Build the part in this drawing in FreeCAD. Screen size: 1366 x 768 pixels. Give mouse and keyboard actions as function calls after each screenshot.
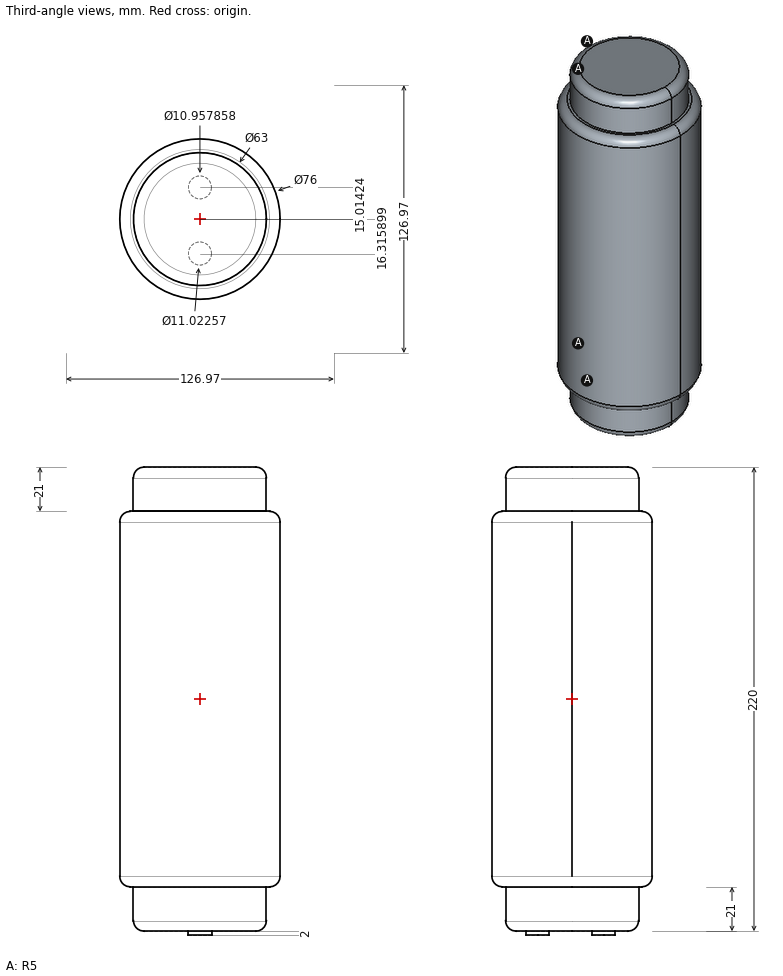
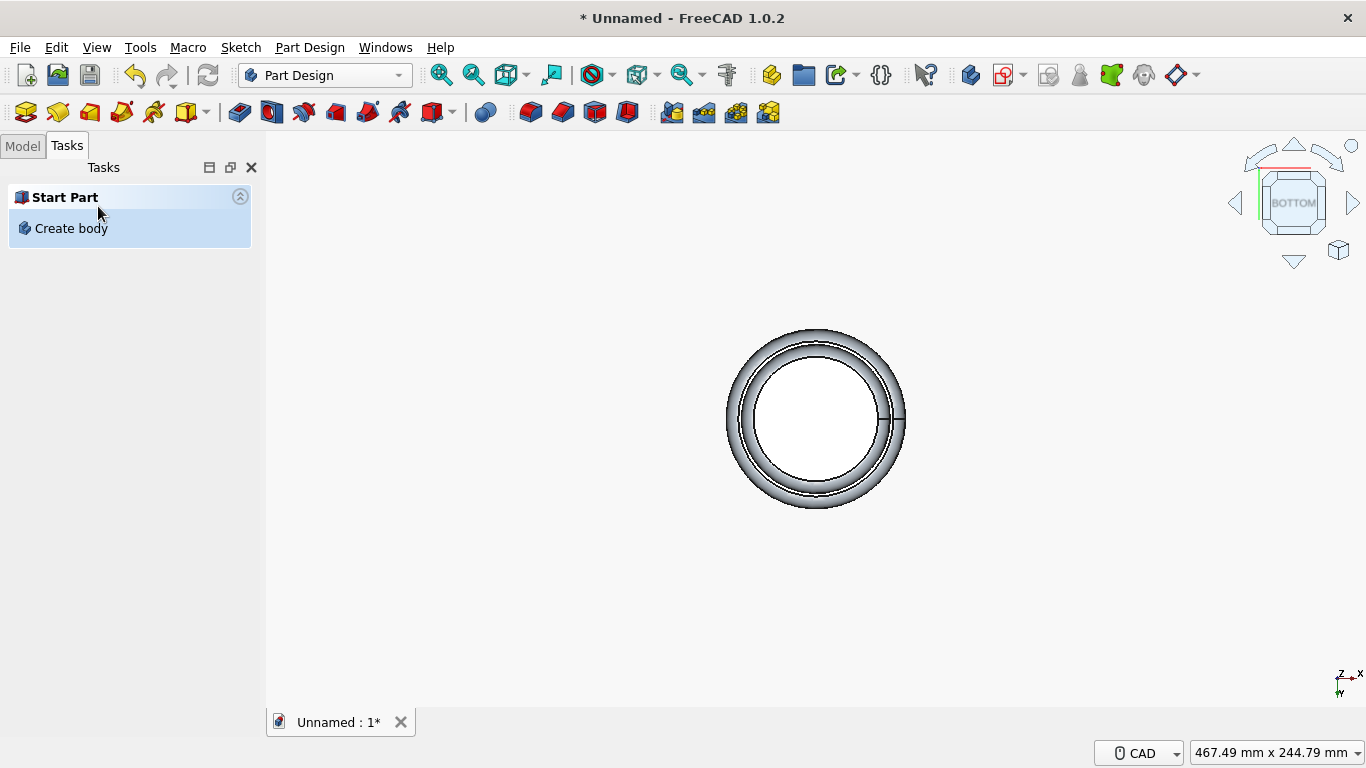
key(v)
key(f)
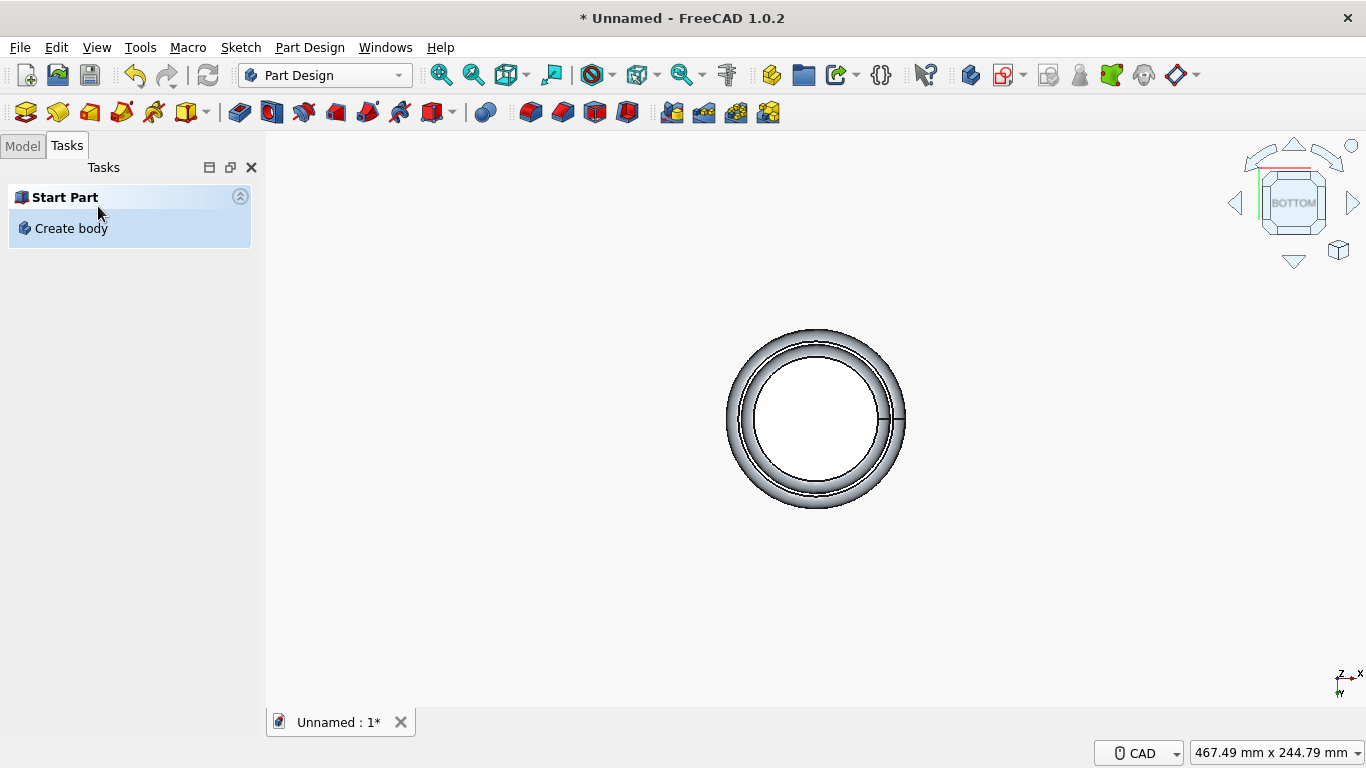
click(816, 418)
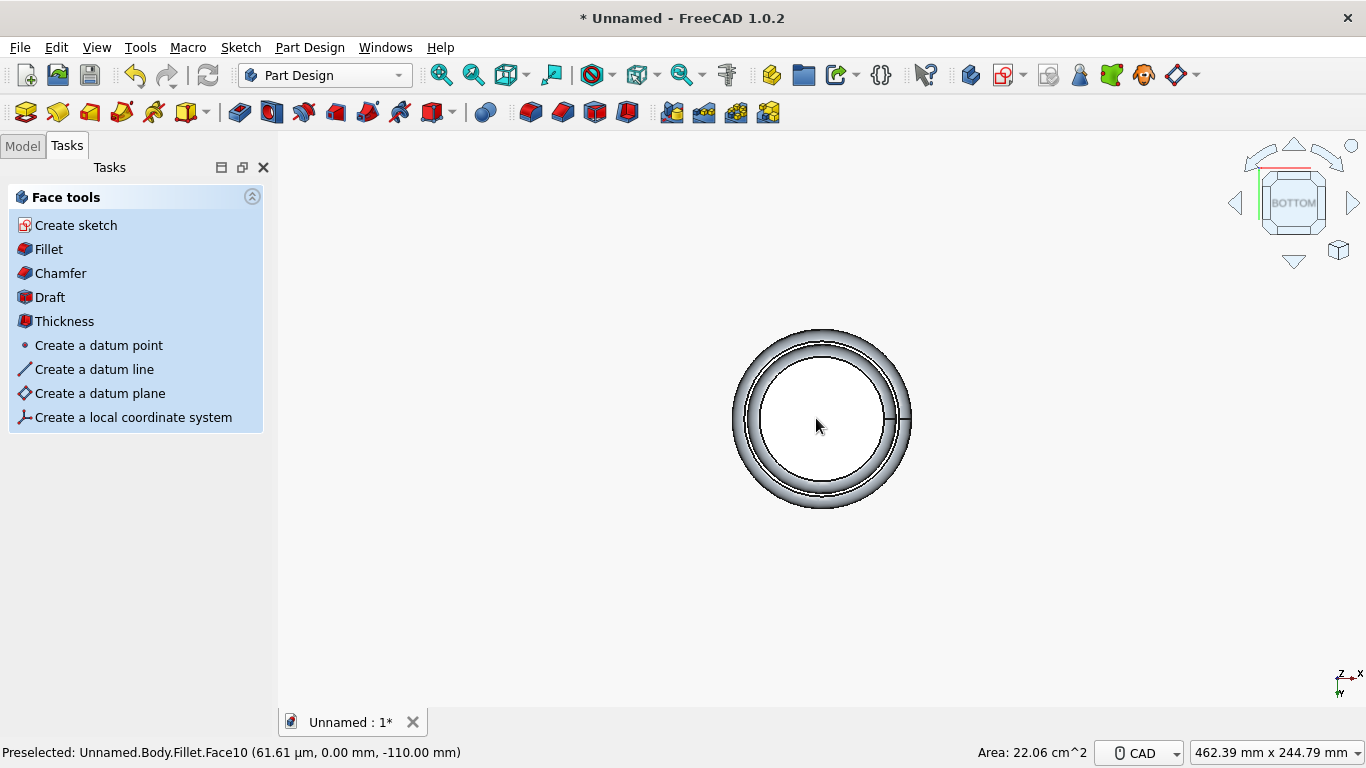
click(1004, 76)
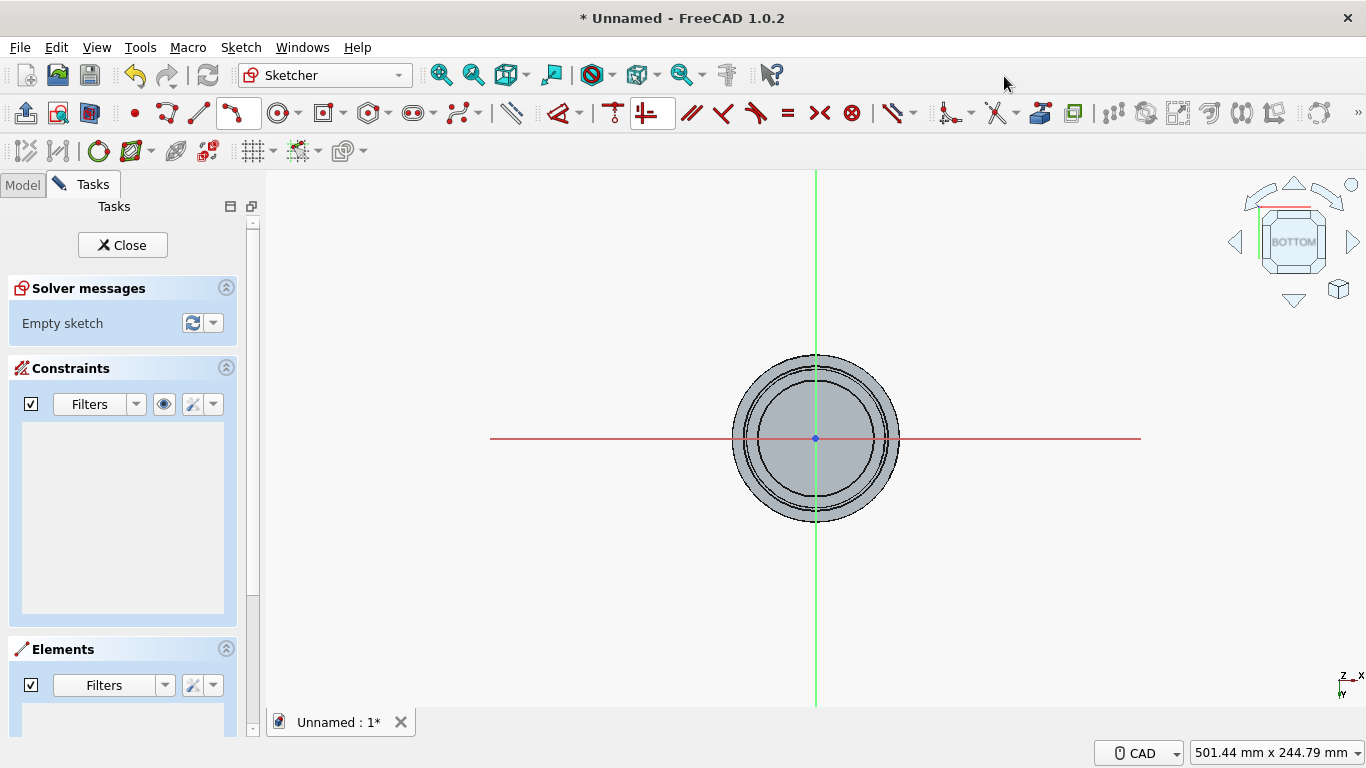
scroll(845, 436, up, 6)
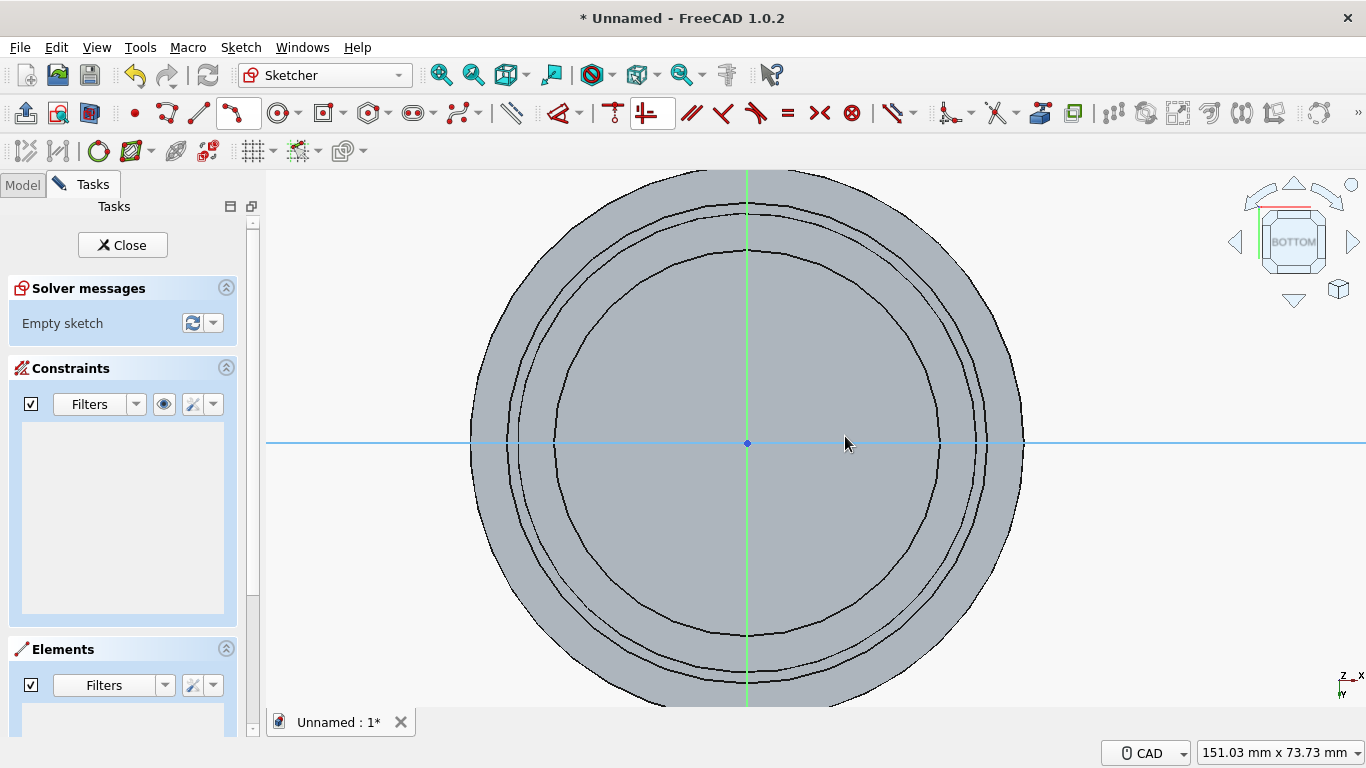
click(278, 114)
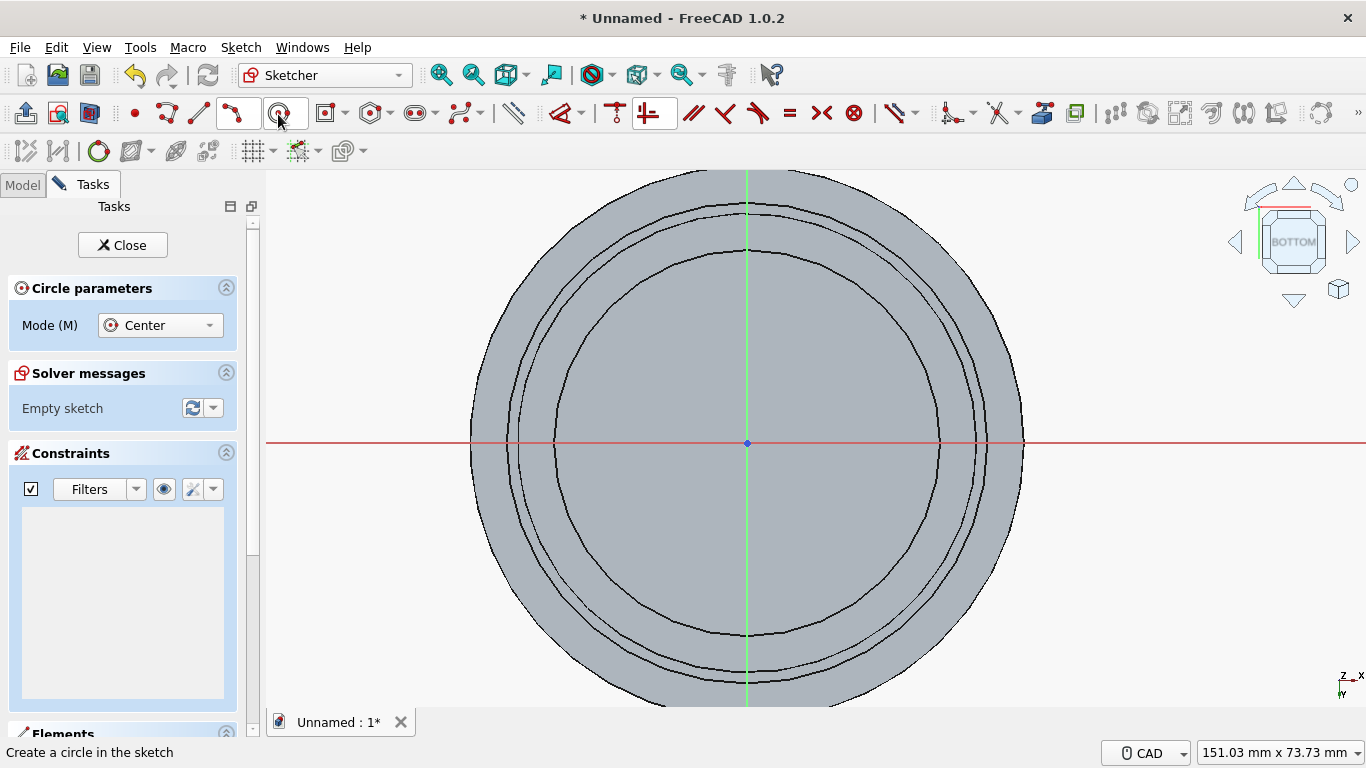
click(747, 553)
move(775, 524)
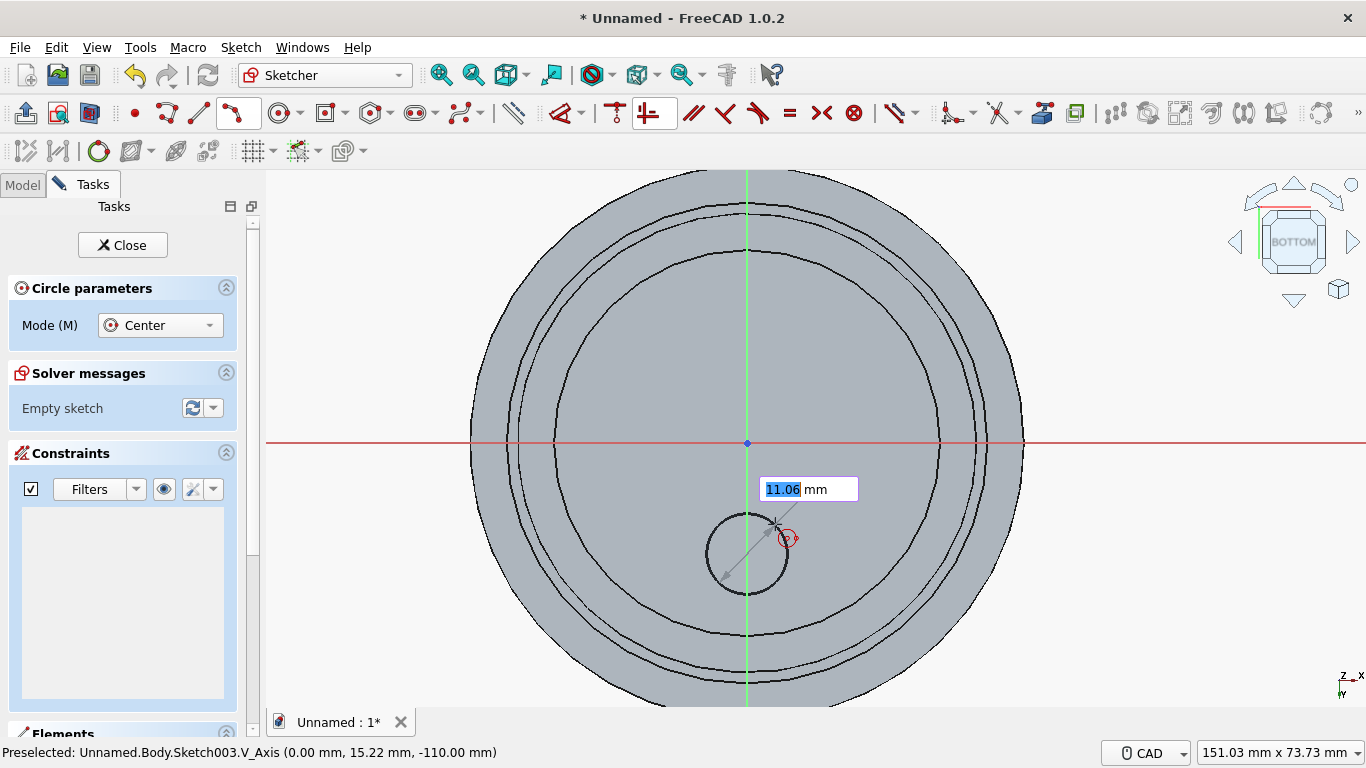
text(10.957858)
key(Return)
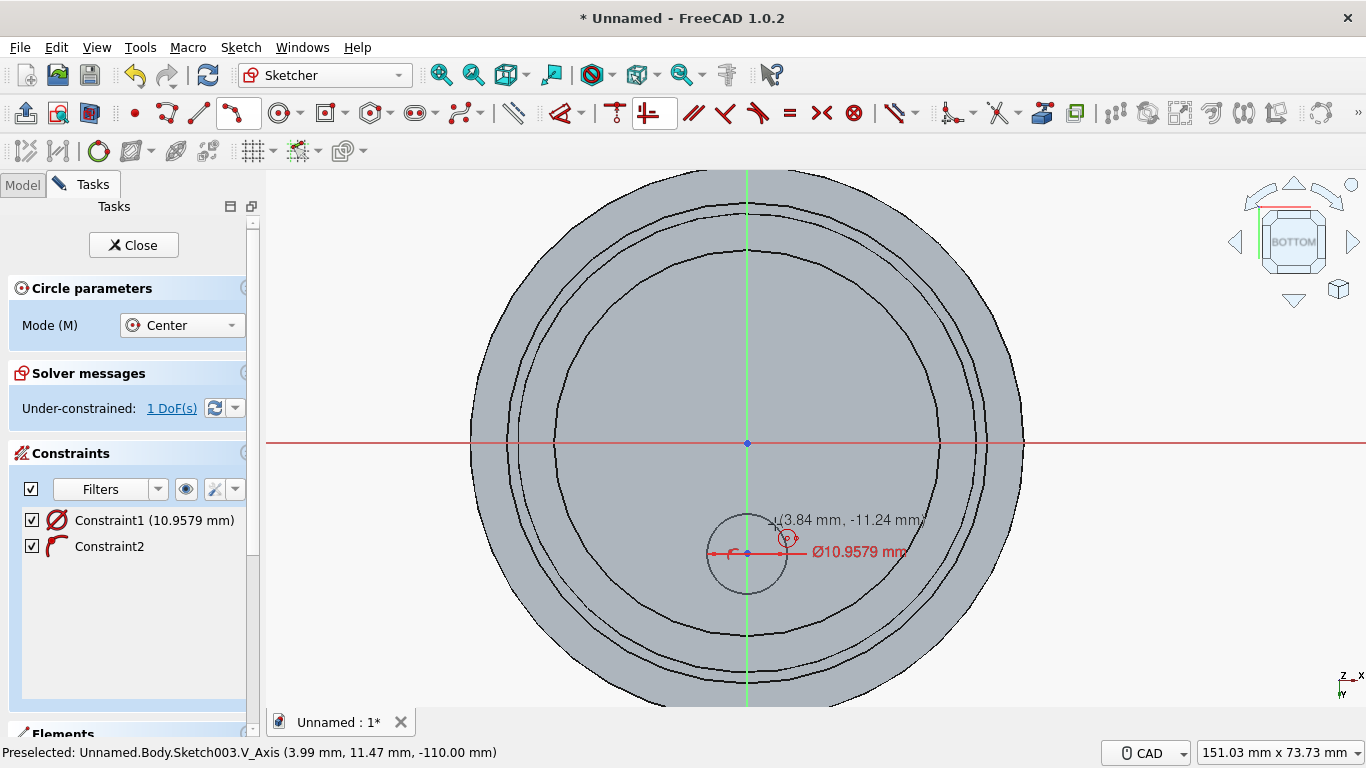
click(747, 324)
move(775, 296)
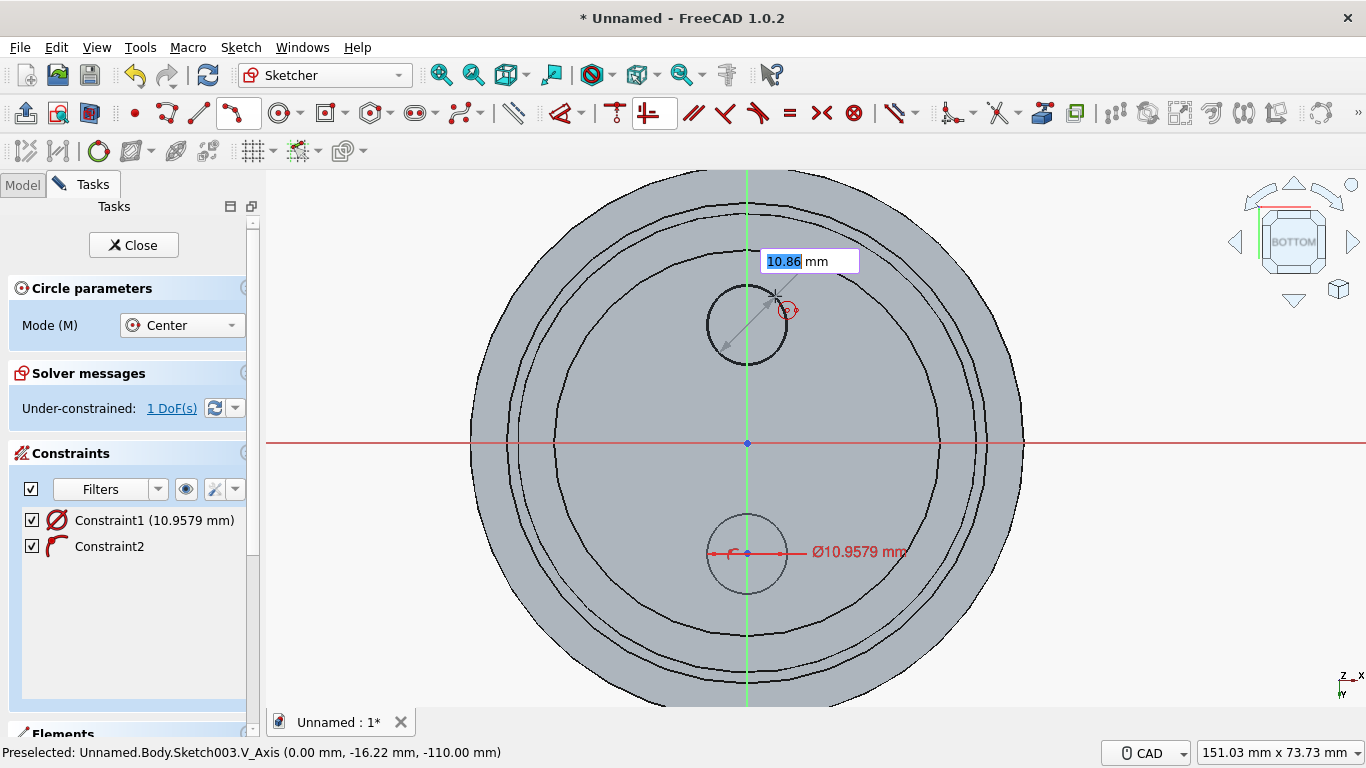
text(11.02257)
key(Return)
key(Escape)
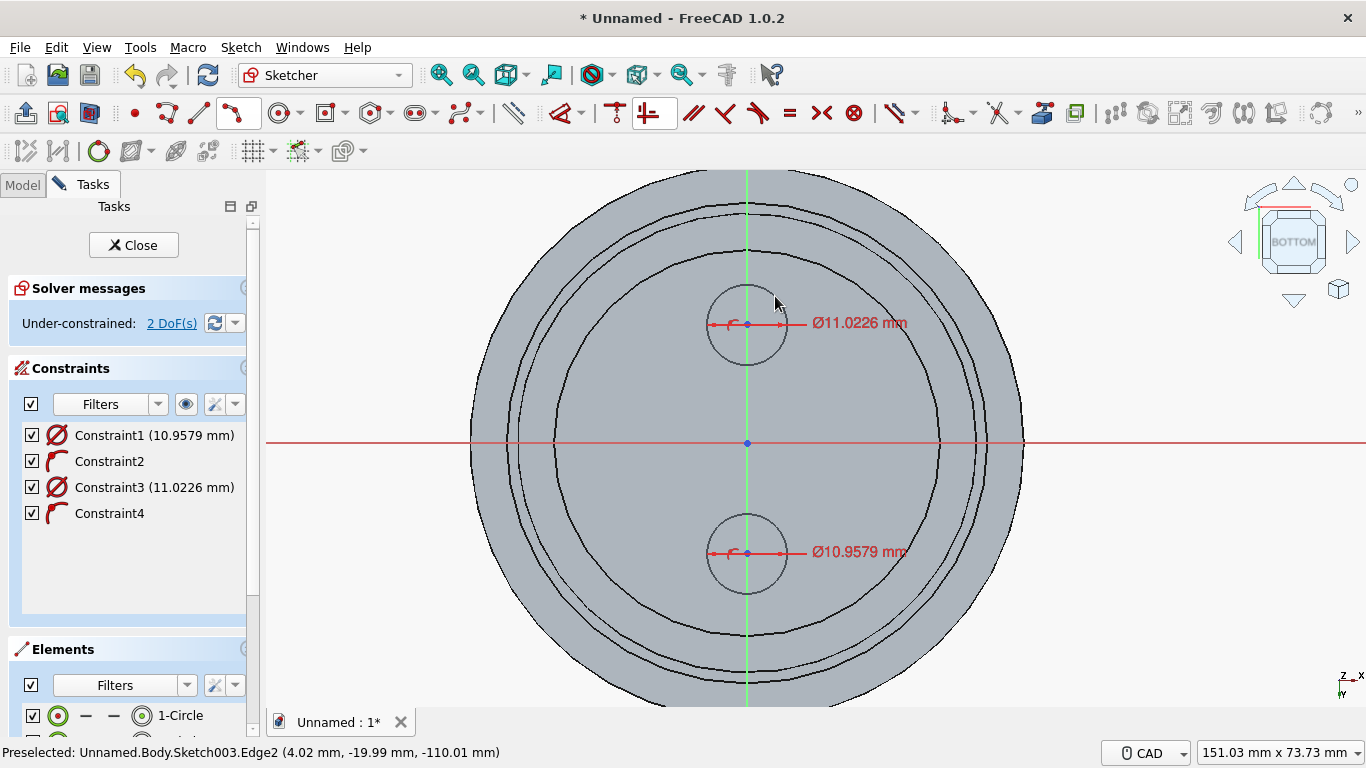
click(560, 114)